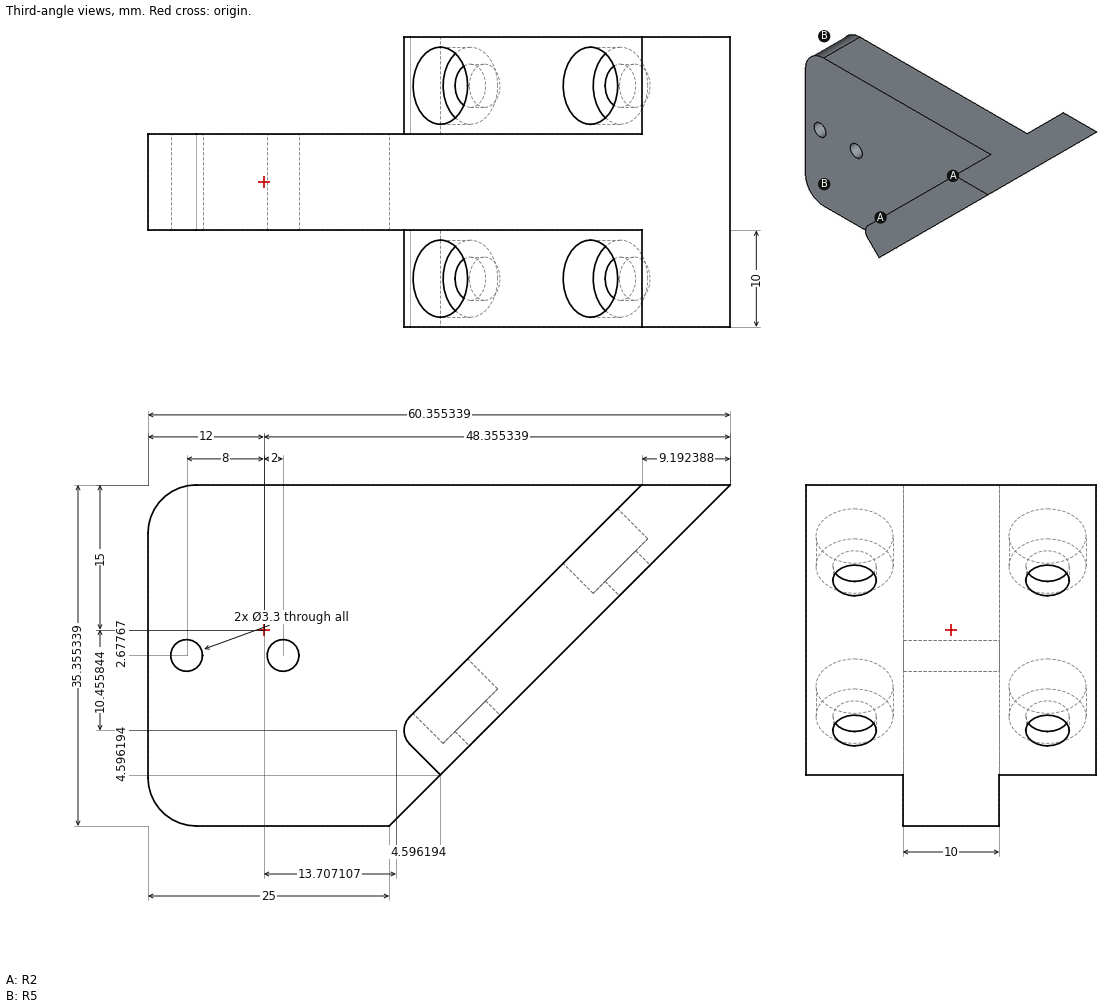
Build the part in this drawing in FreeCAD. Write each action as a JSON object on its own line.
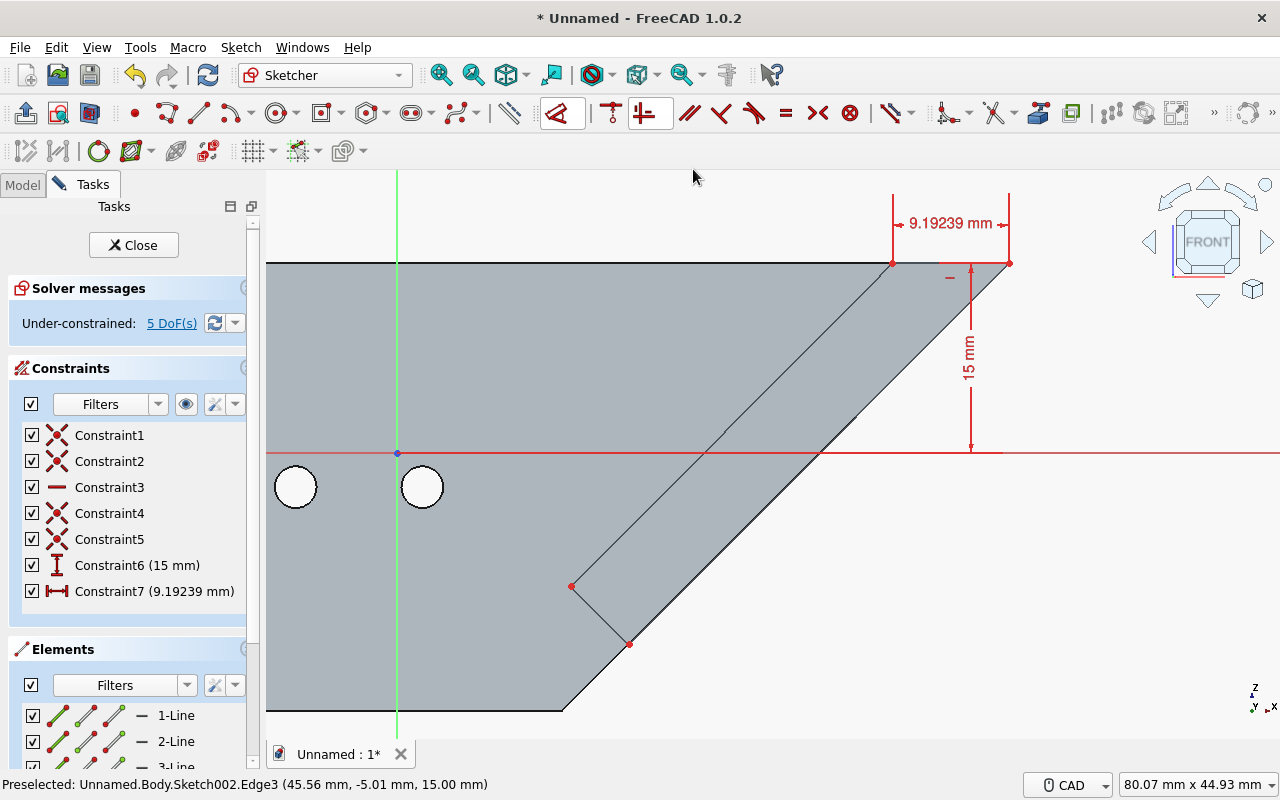
{"action": "left_click", "coordinate": [588, 604]}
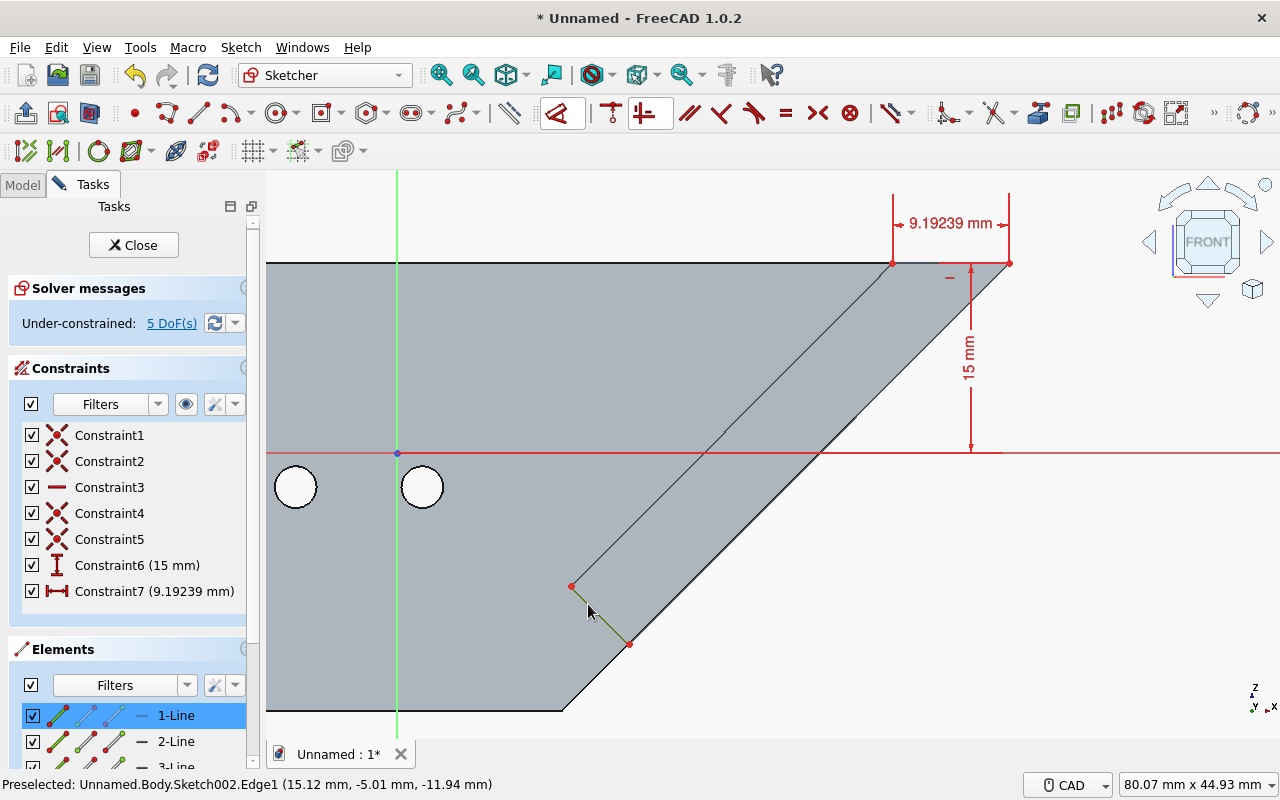
{"action": "left_click", "coordinate": [580, 114]}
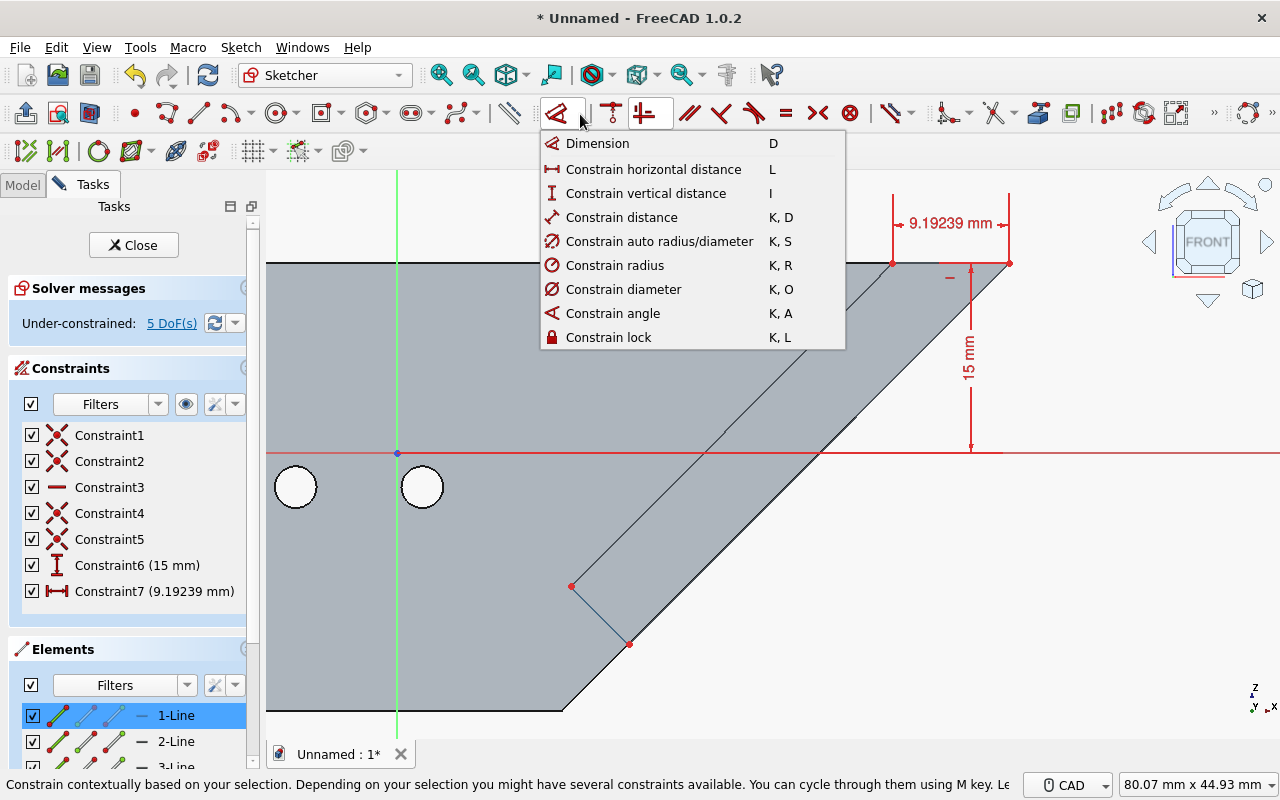
{"action": "left_click", "coordinate": [693, 169]}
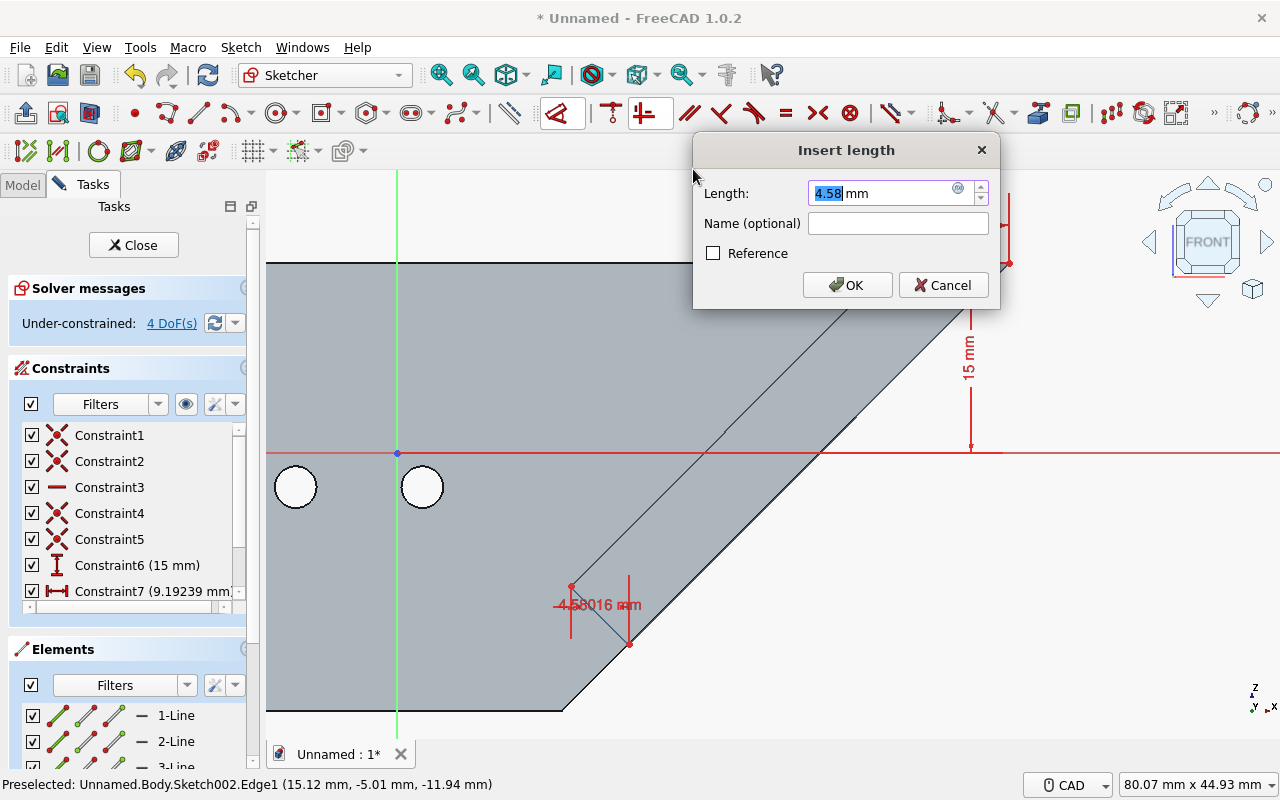
{"action": "type", "text": "4.596194"}
{"action": "key", "text": "Return"}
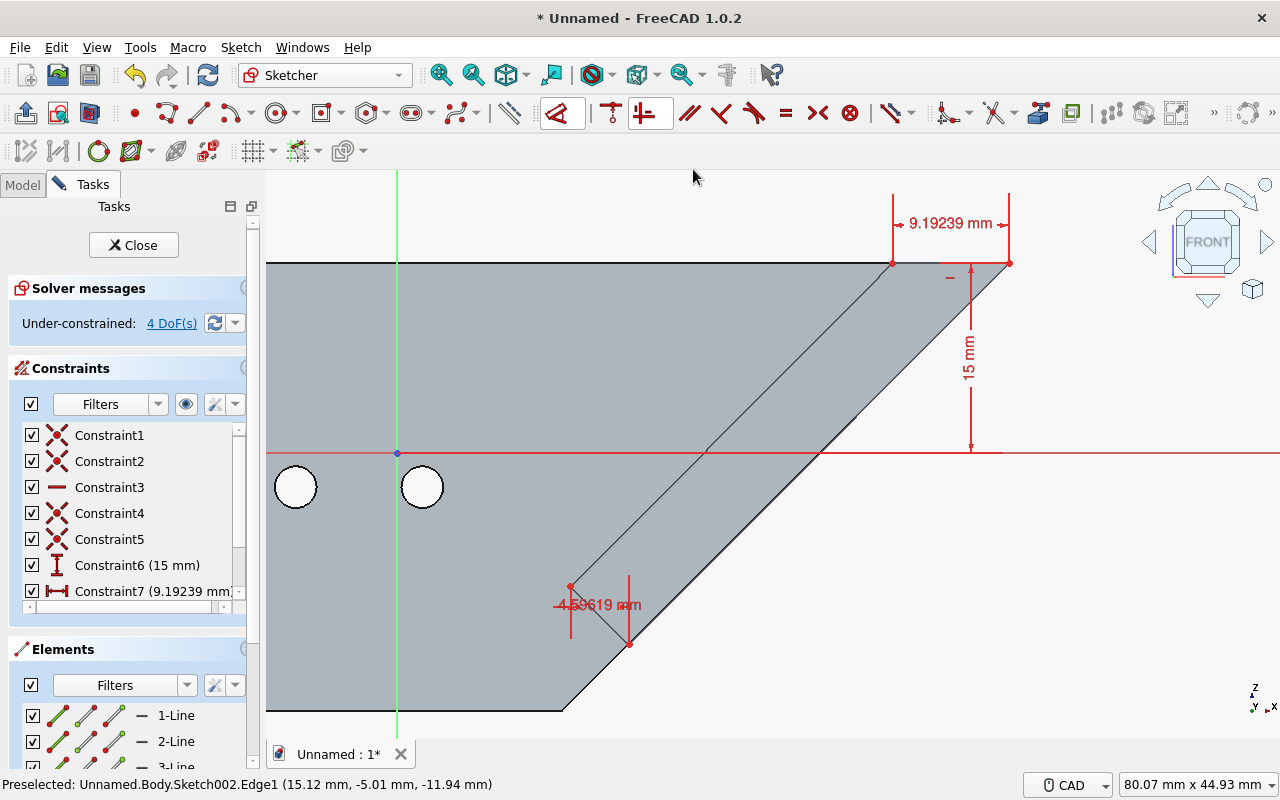
{"action": "left_click", "coordinate": [612, 628]}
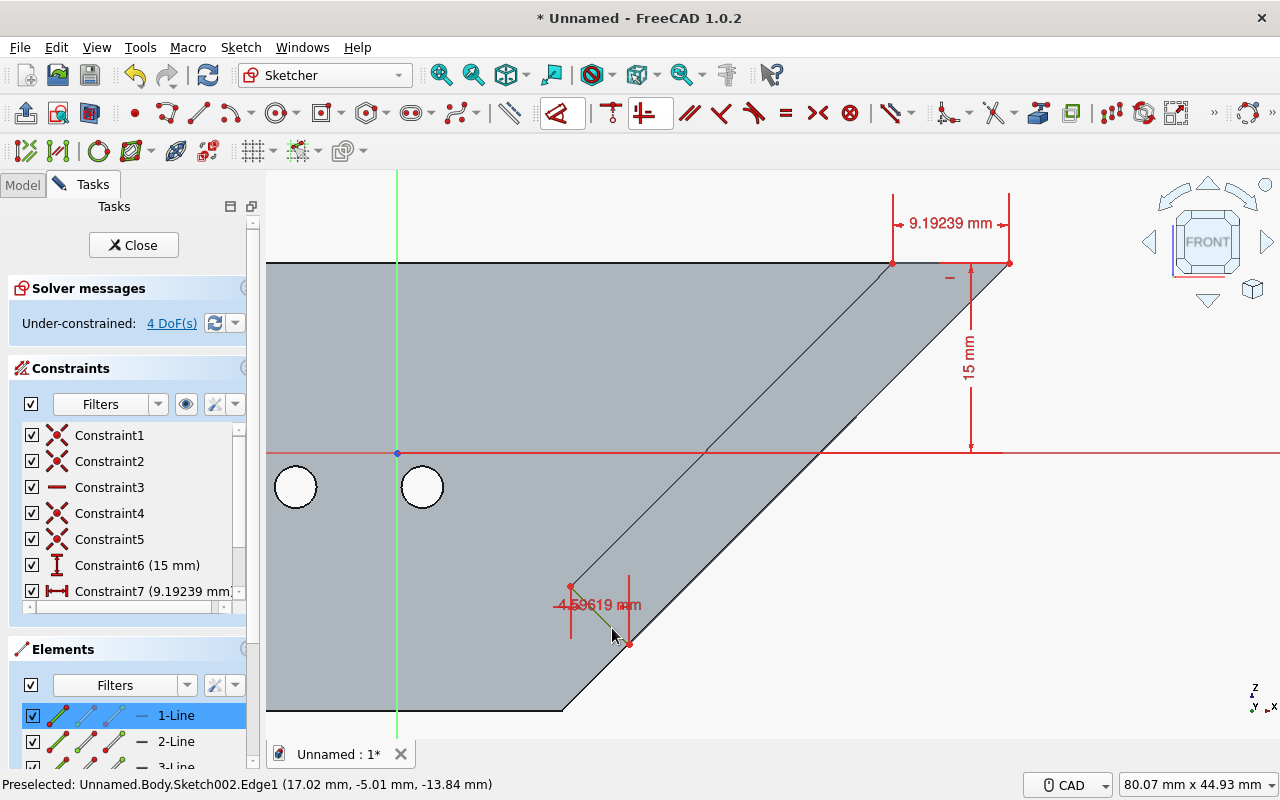
{"action": "left_click", "coordinate": [580, 114]}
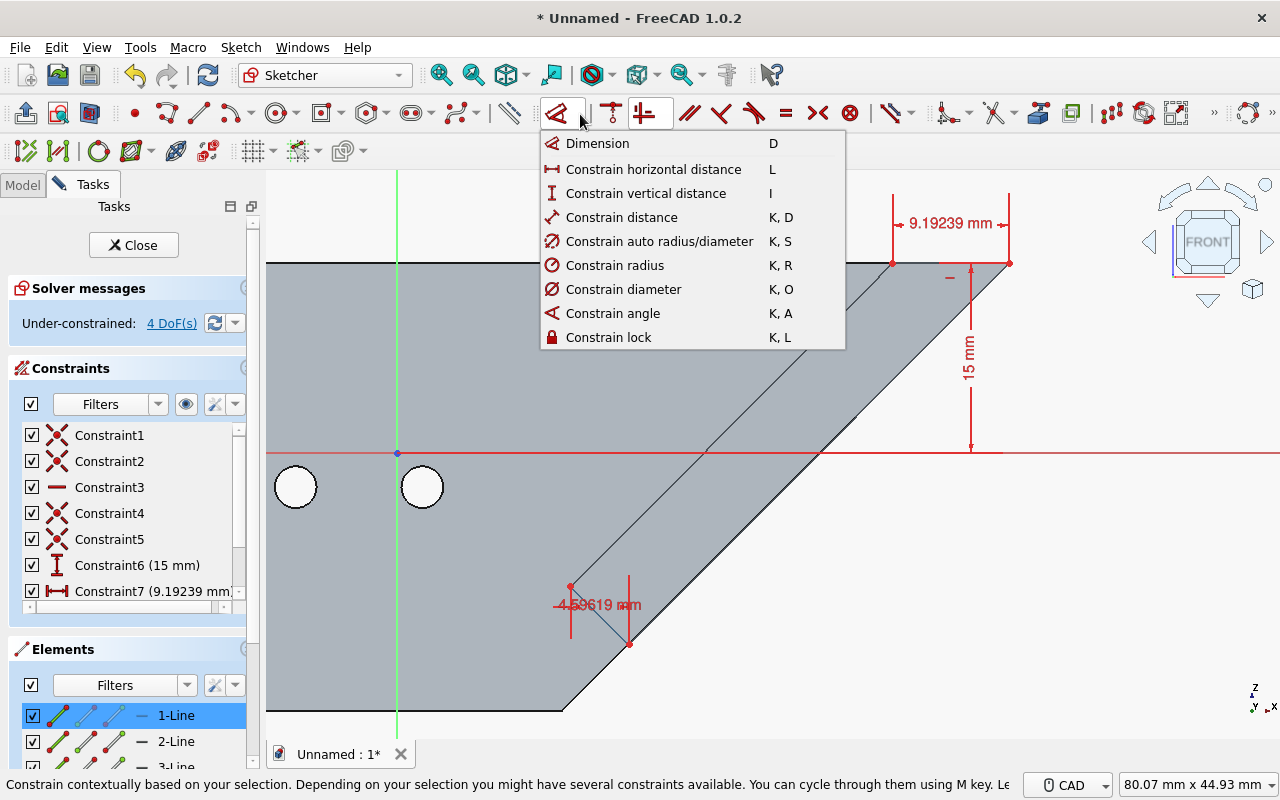
{"action": "left_click", "coordinate": [693, 193]}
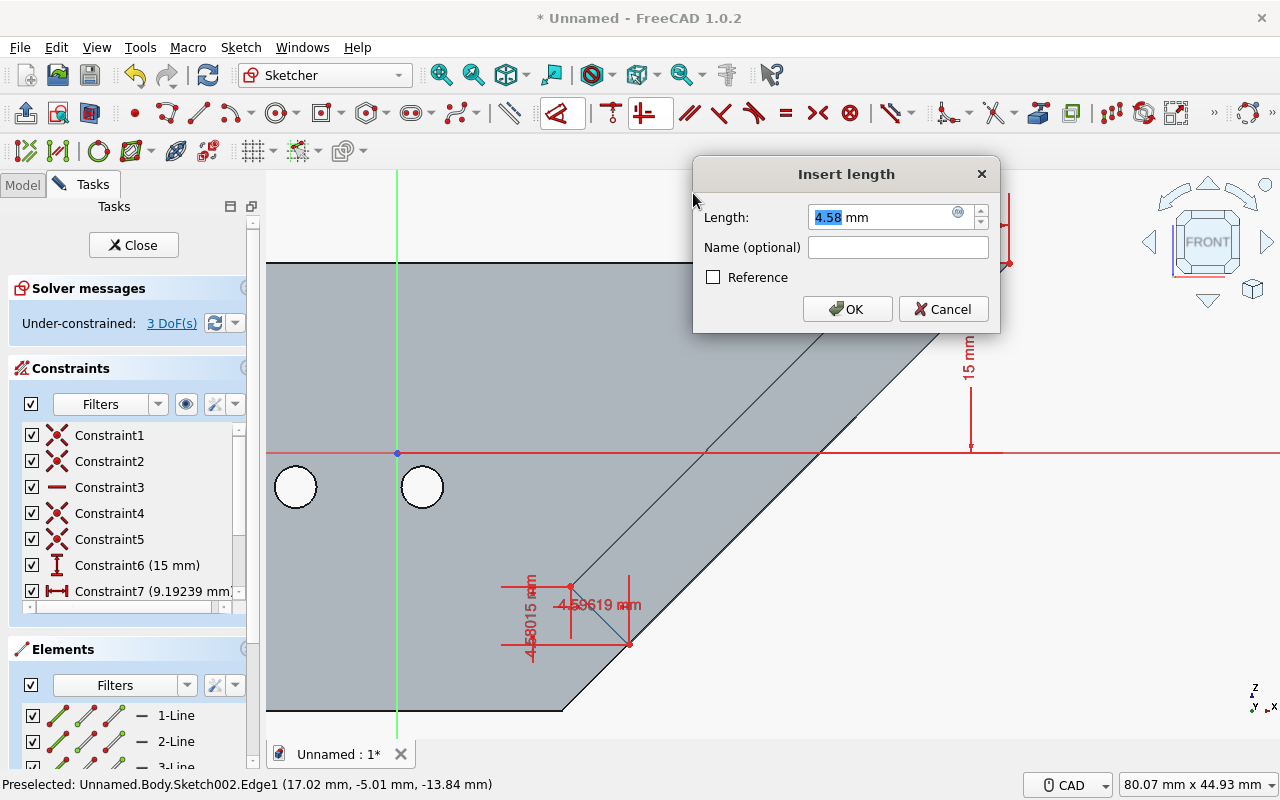
{"action": "type", "text": "4.596194"}
{"action": "key", "text": "Return"}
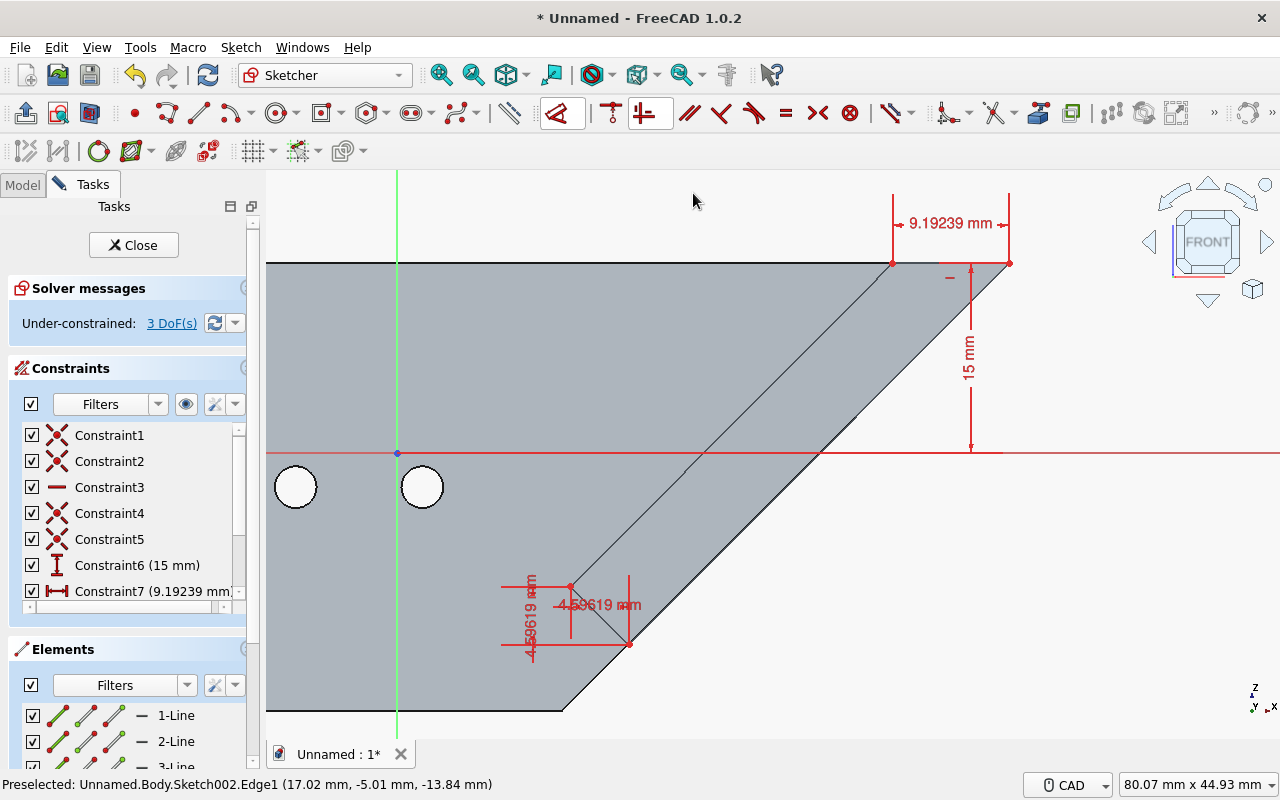
{"action": "left_click", "coordinate": [571, 587]}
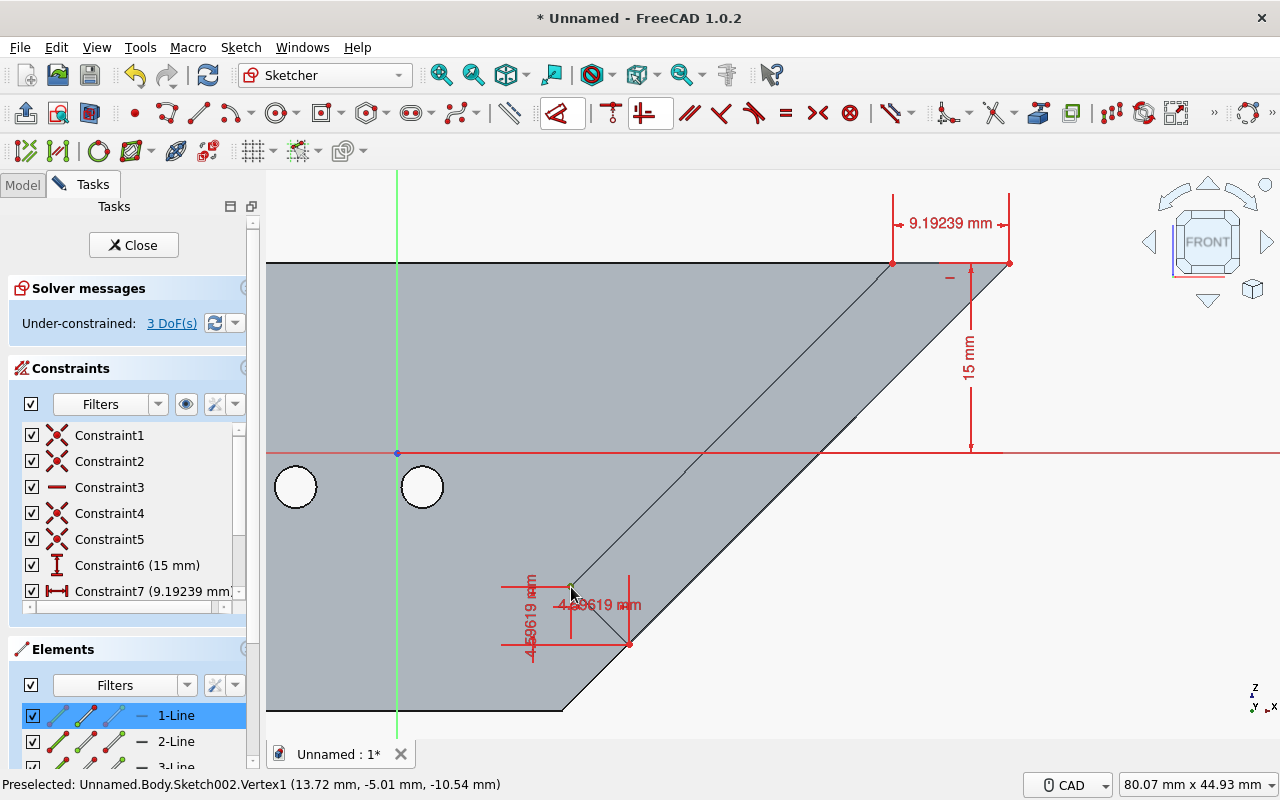
{"action": "left_click", "coordinate": [580, 114]}